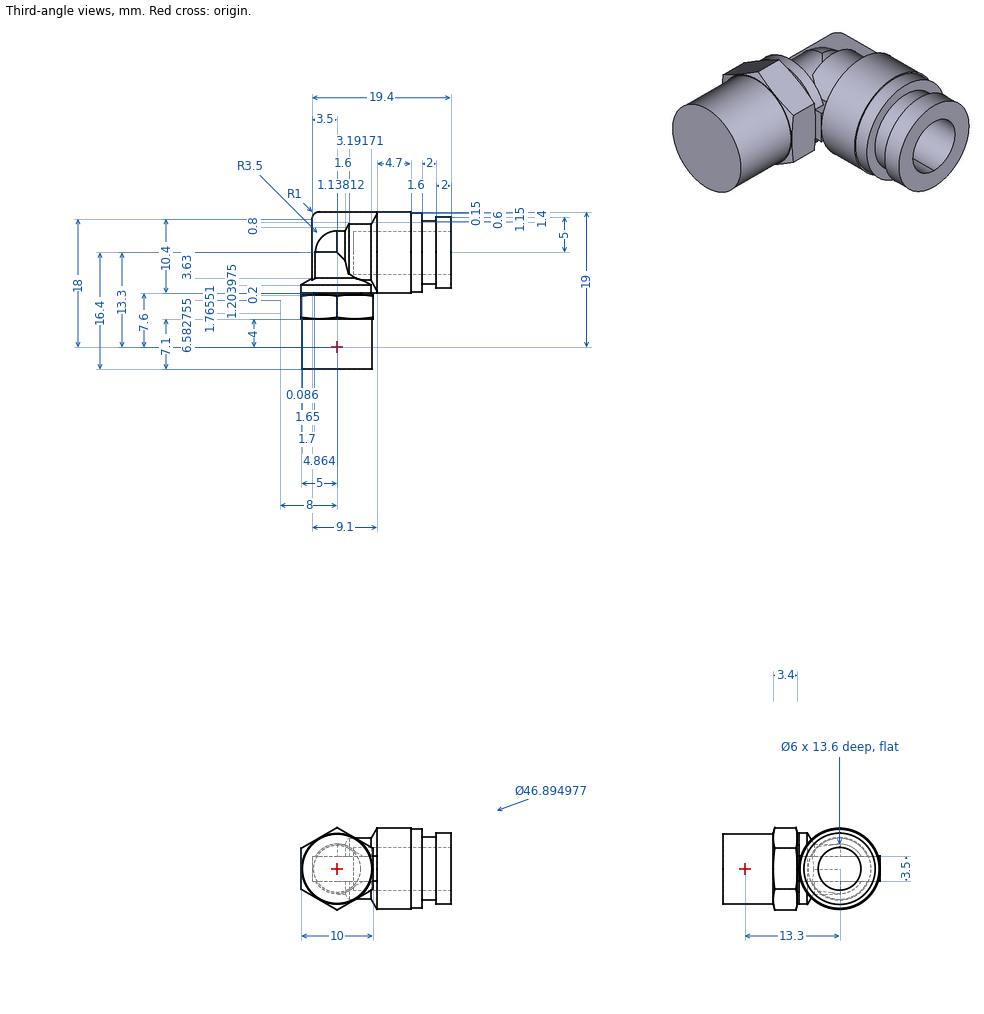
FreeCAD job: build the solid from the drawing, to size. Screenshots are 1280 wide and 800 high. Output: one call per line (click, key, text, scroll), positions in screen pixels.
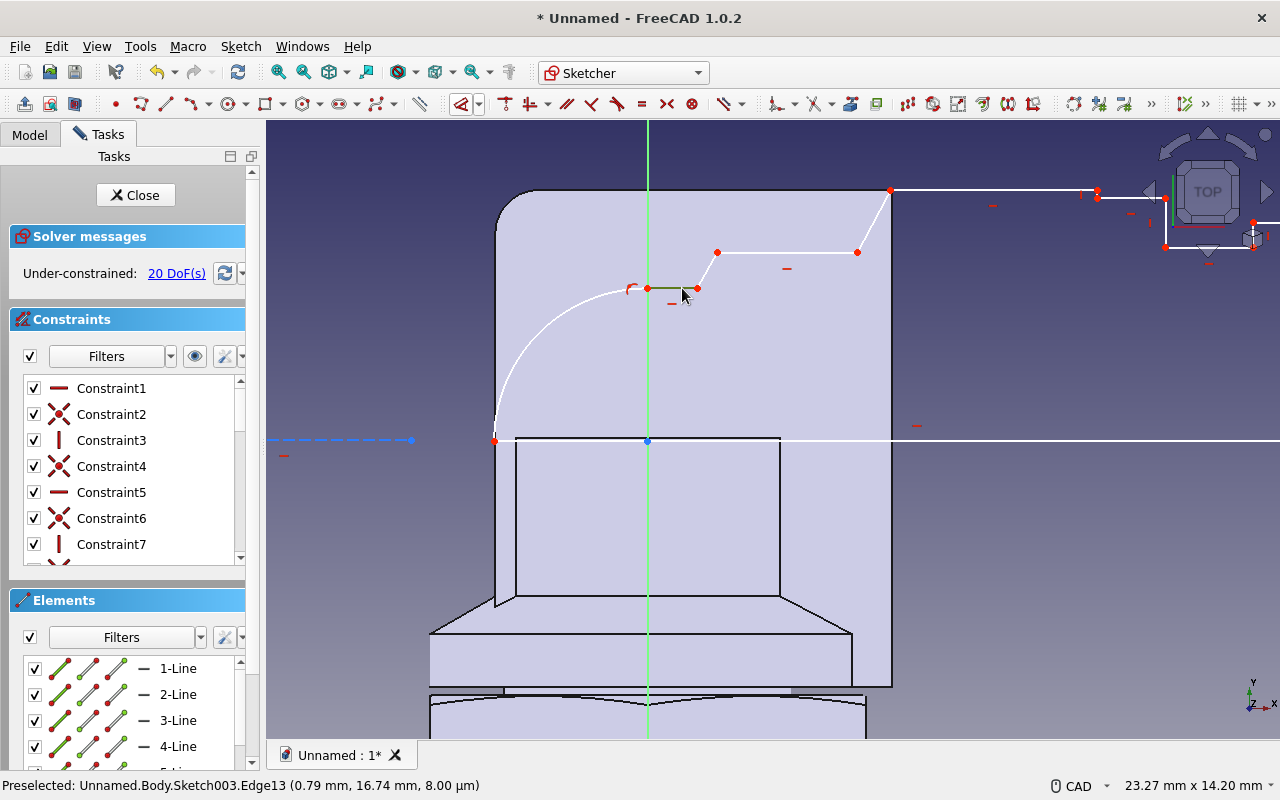
click(578, 305)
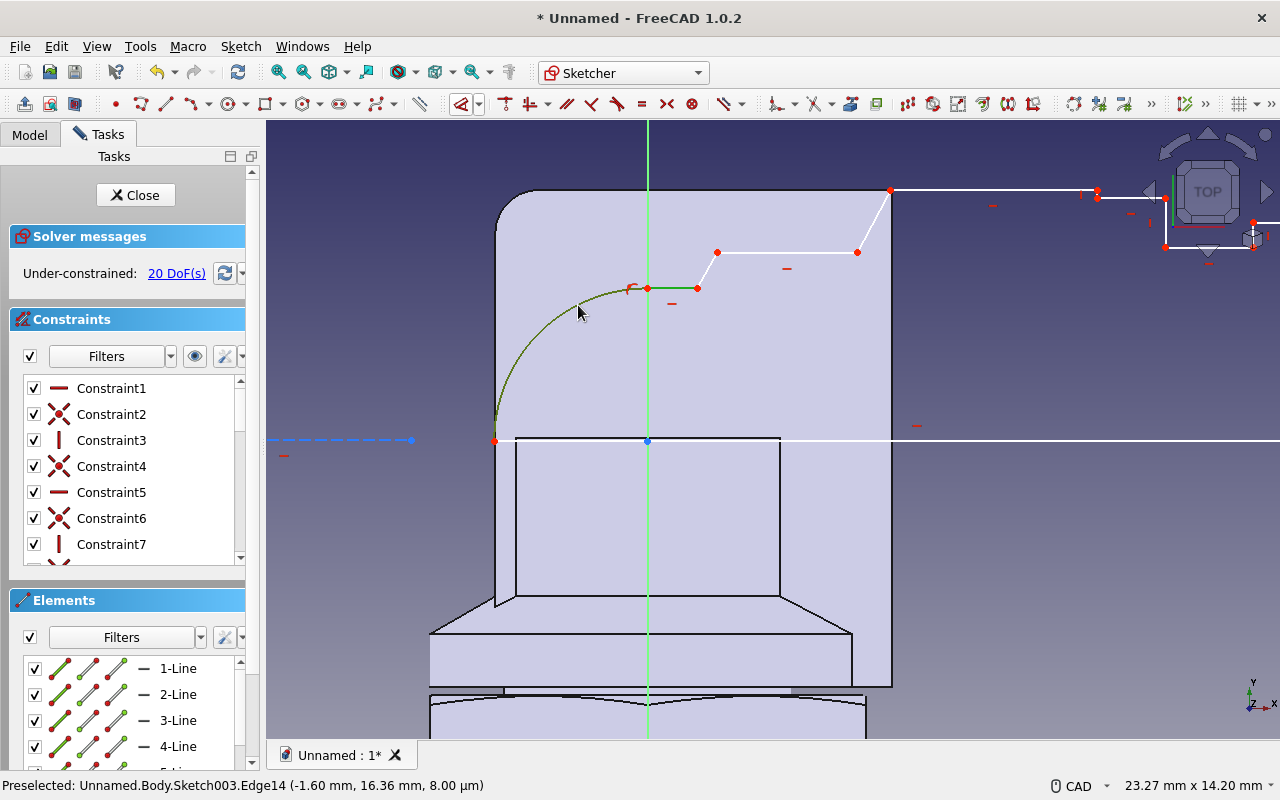
key(t)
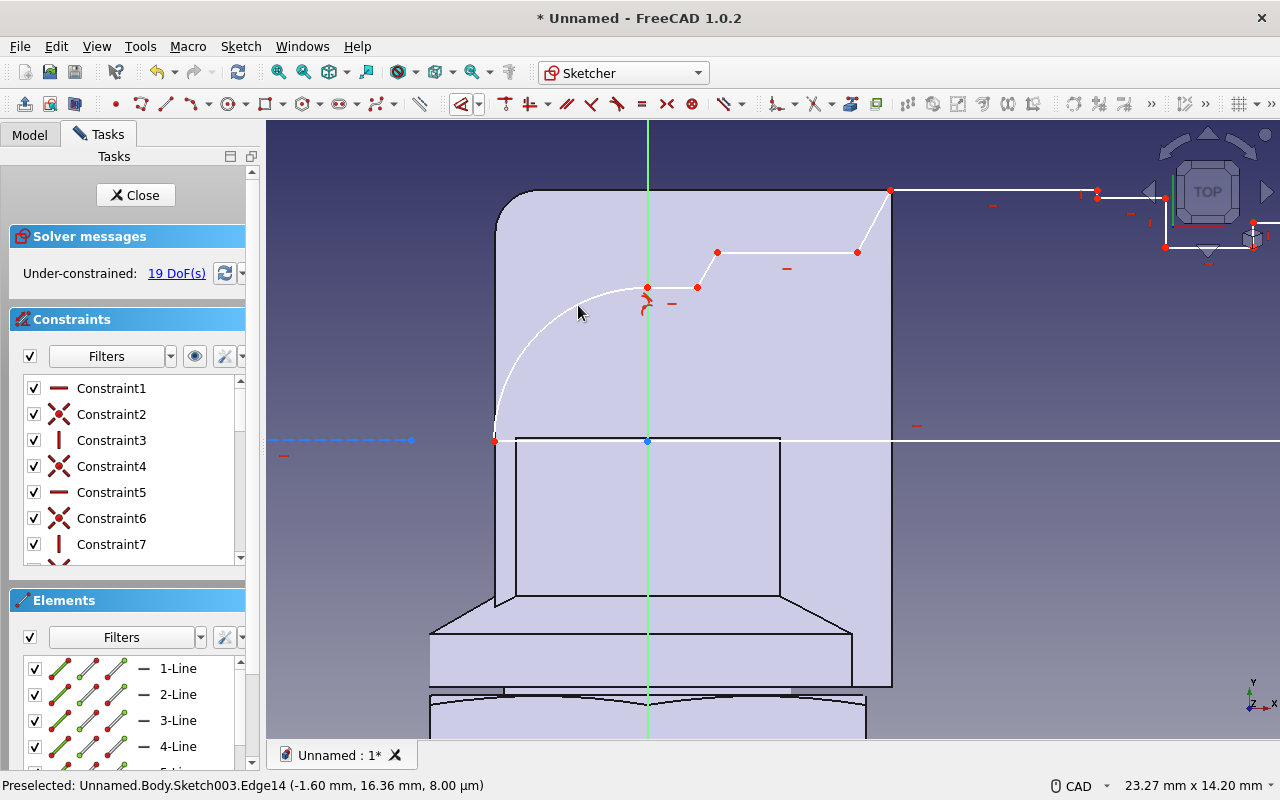
click(578, 304)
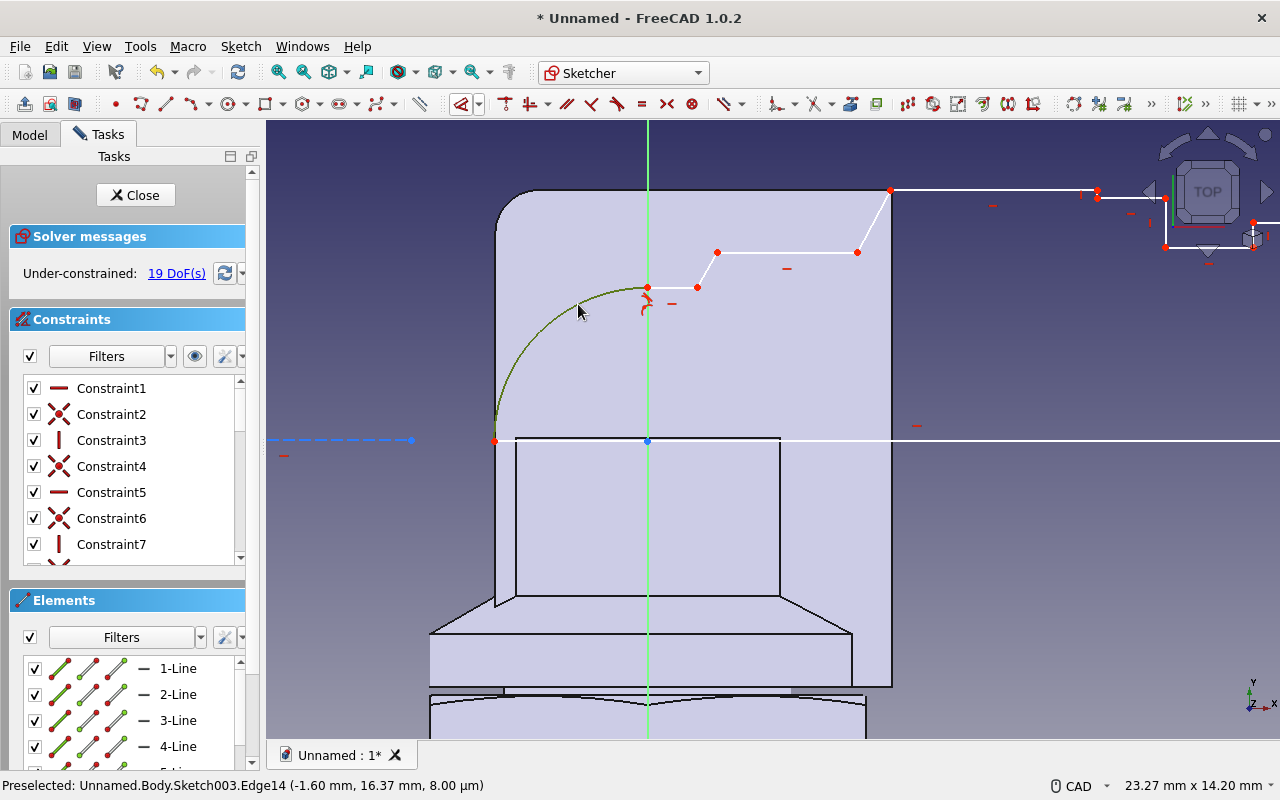
key(k)
key(r)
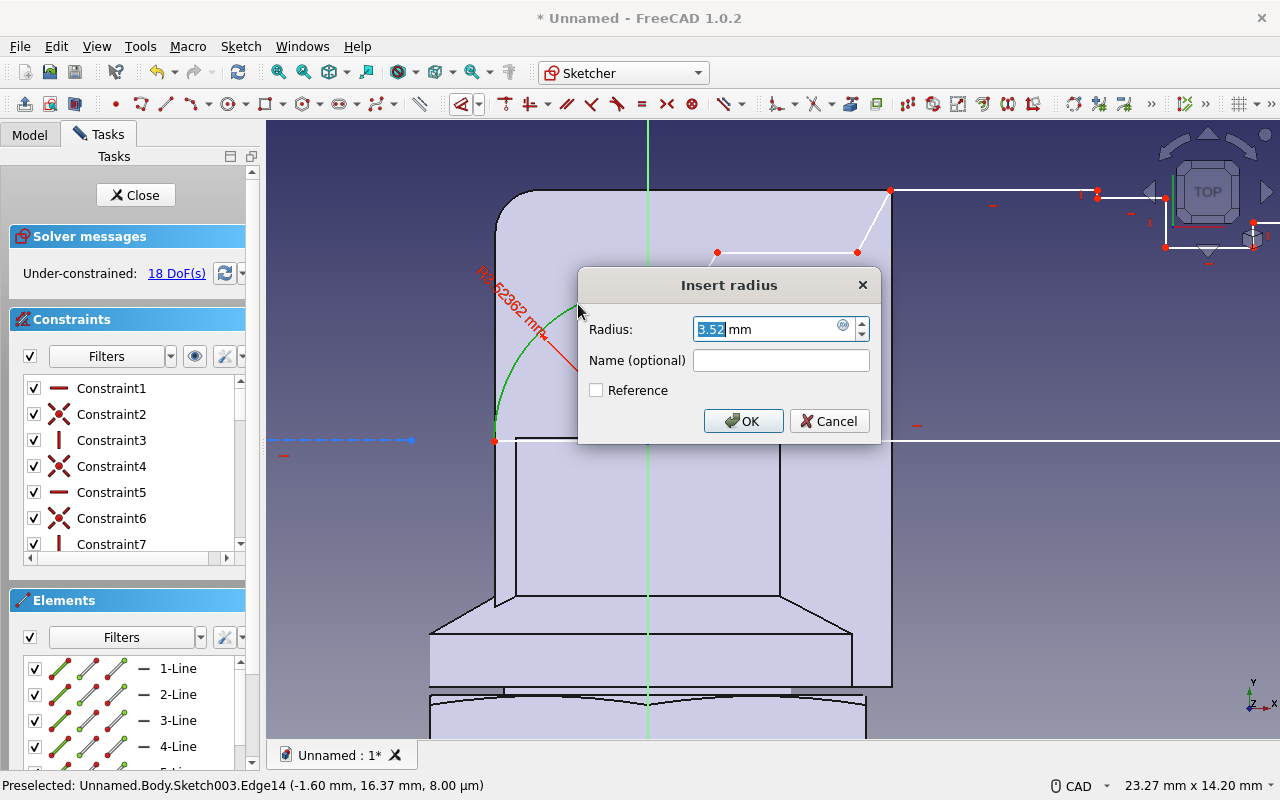
text(3.5)
key(Return)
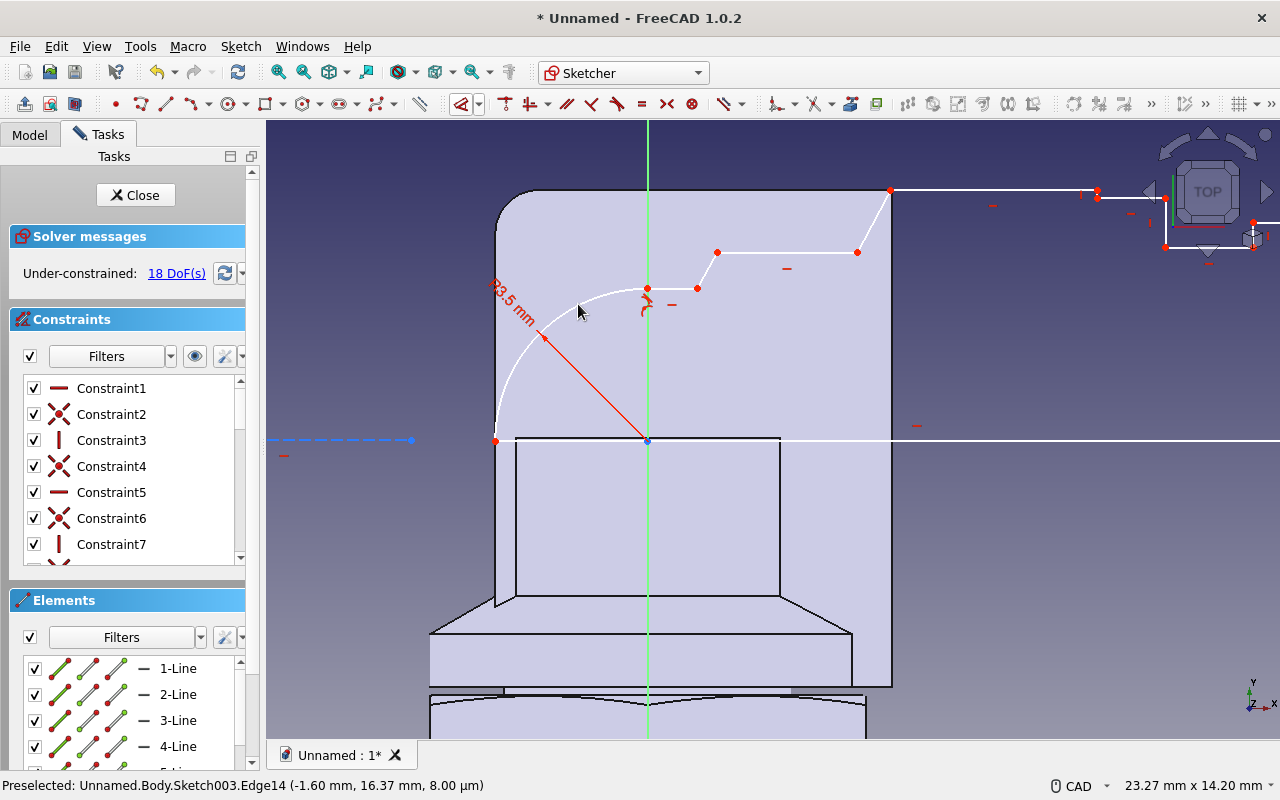
scroll(668, 287, down, 4)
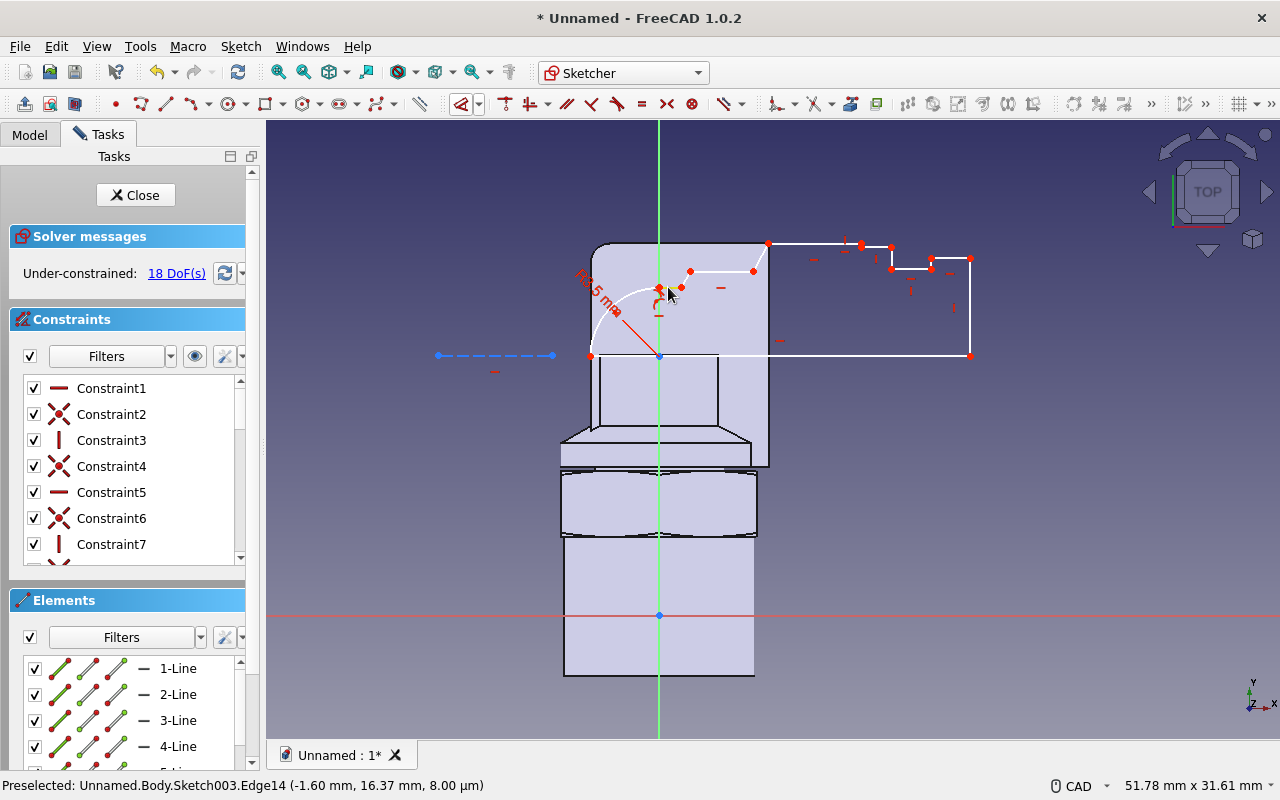
click(970, 327)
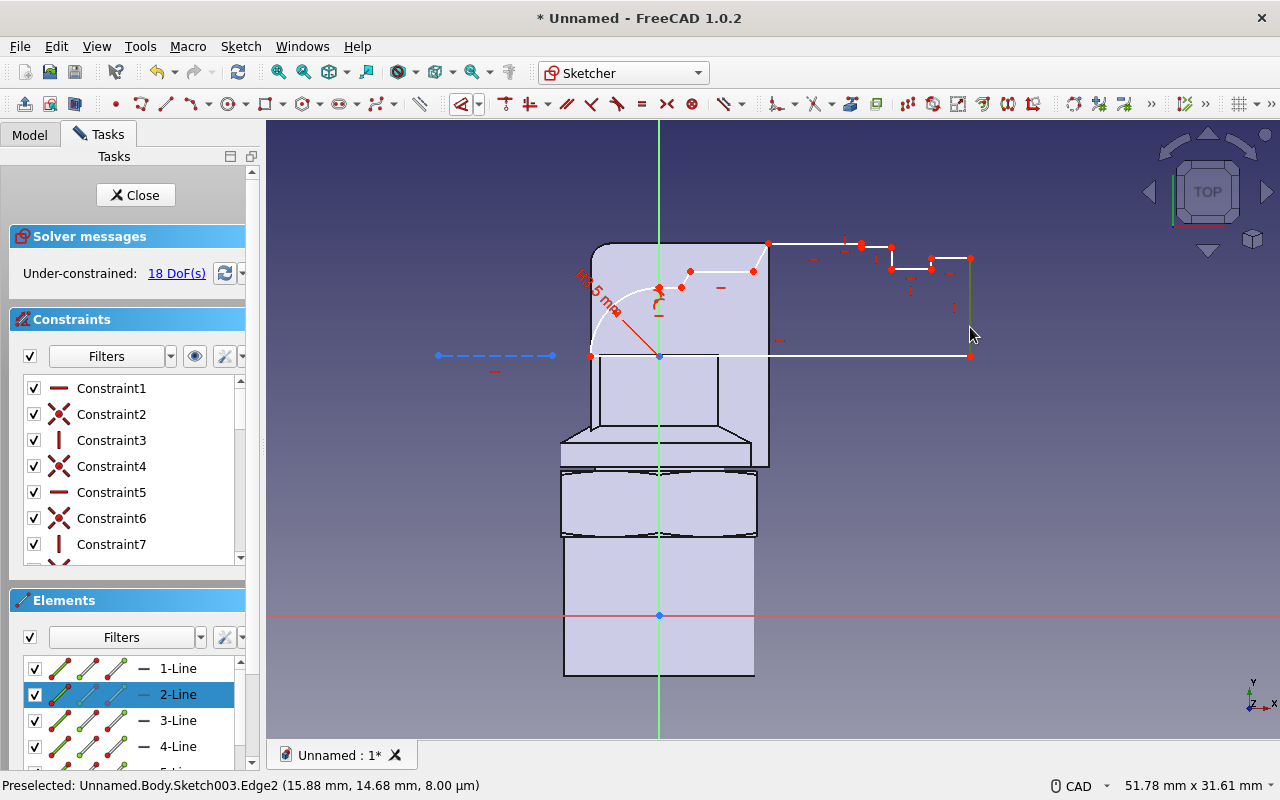
click(478, 104)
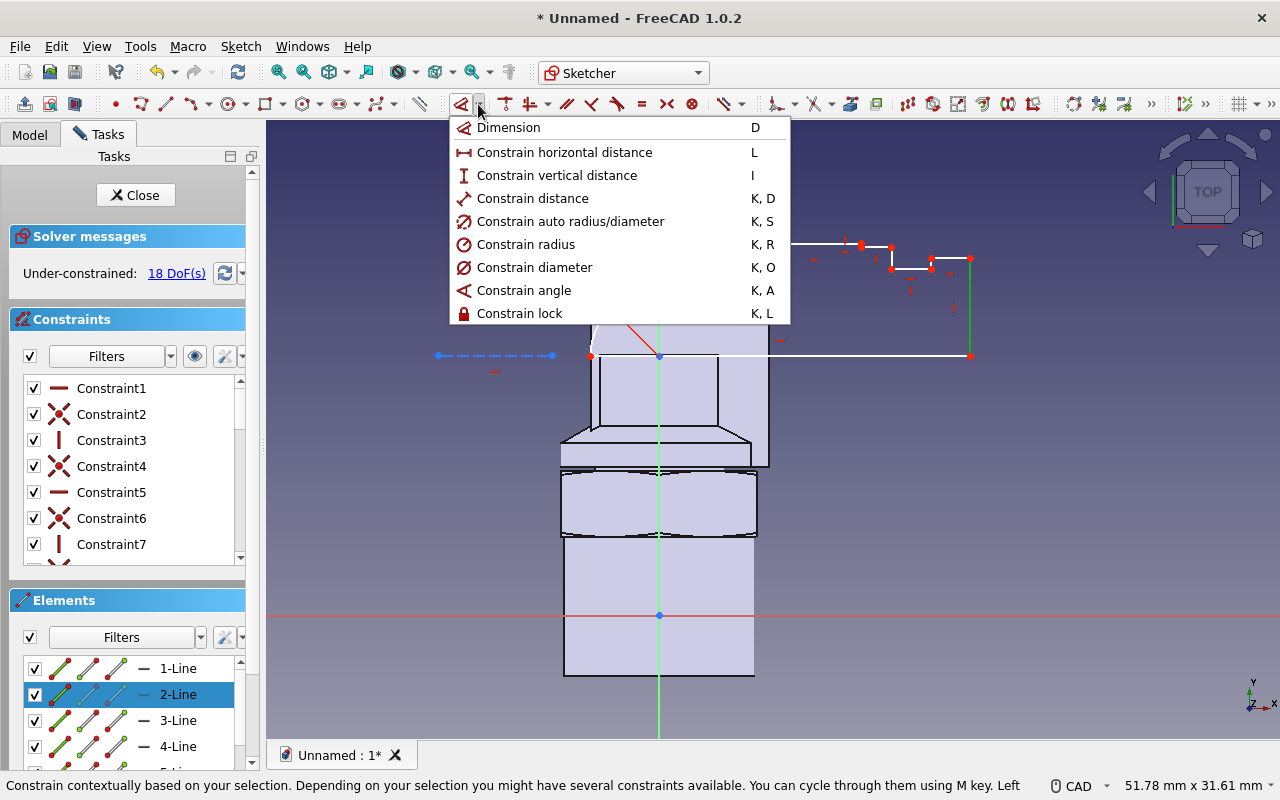
click(620, 176)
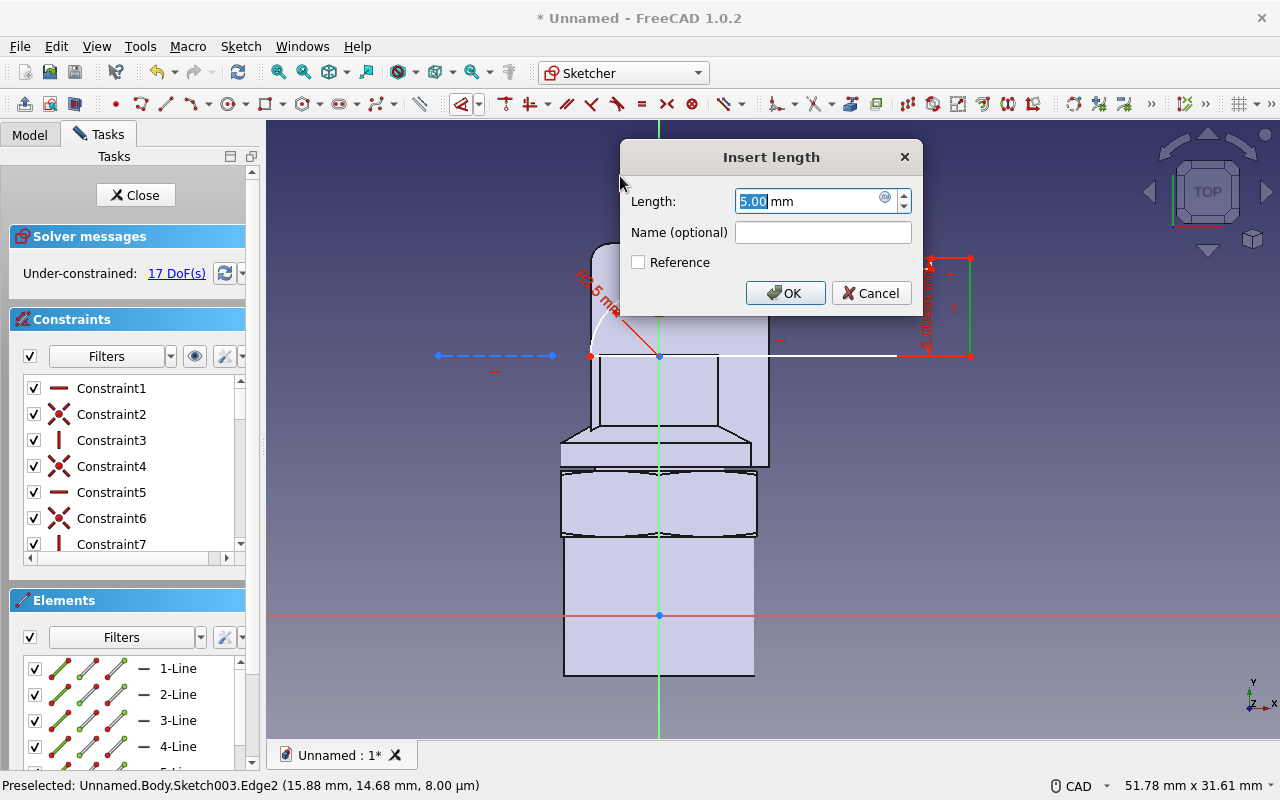
text(5)
key(Return)